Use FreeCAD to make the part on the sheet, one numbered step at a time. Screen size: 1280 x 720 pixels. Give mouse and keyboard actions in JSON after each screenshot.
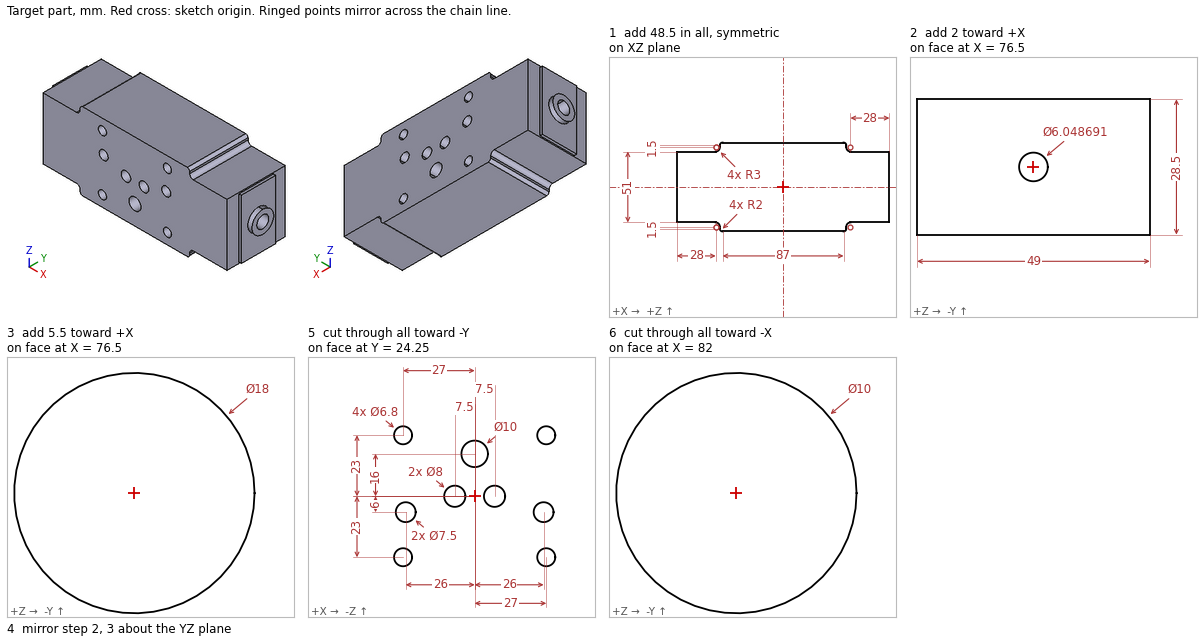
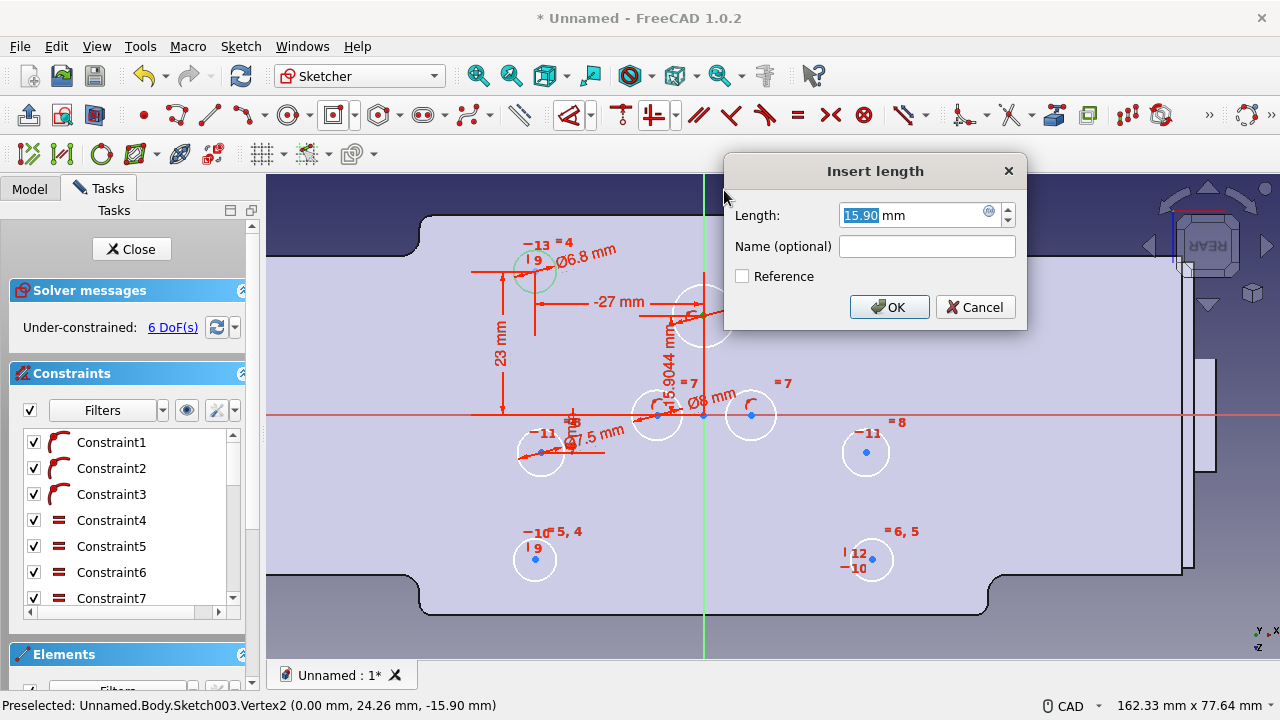
{"action": "type", "text": "16"}
{"action": "key", "text": "Return"}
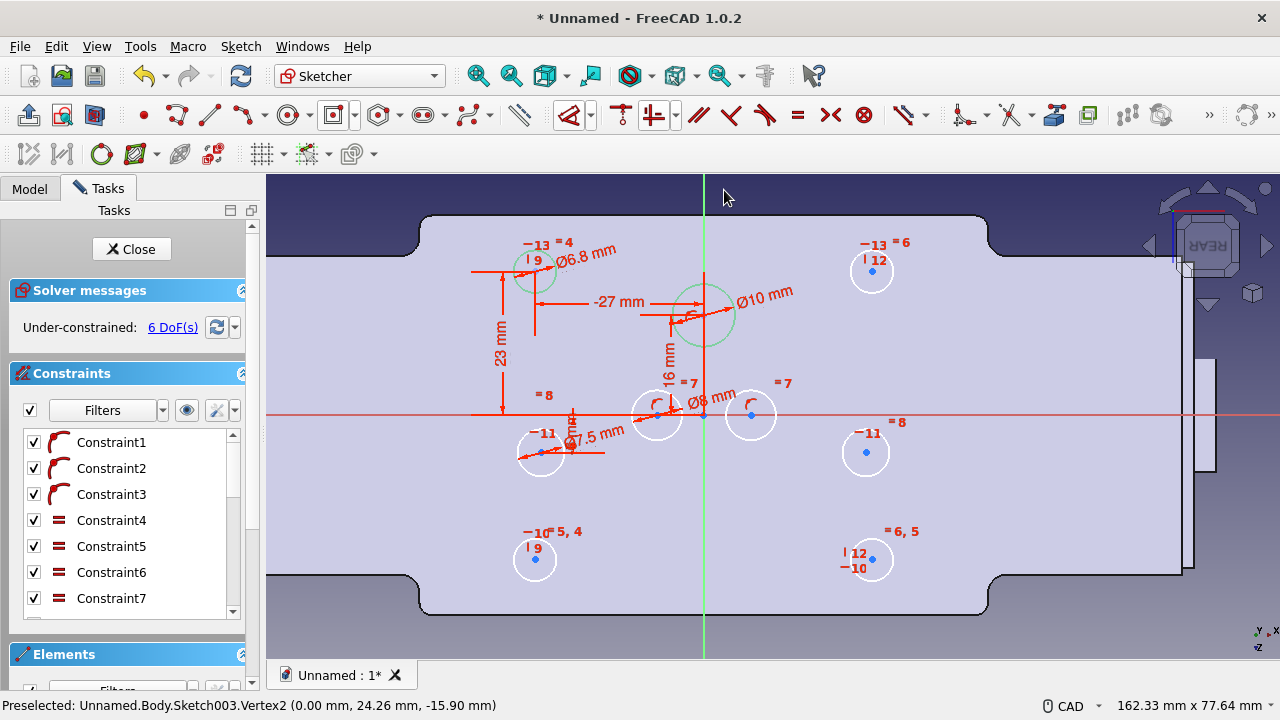
{"action": "left_click", "coordinate": [541, 453]}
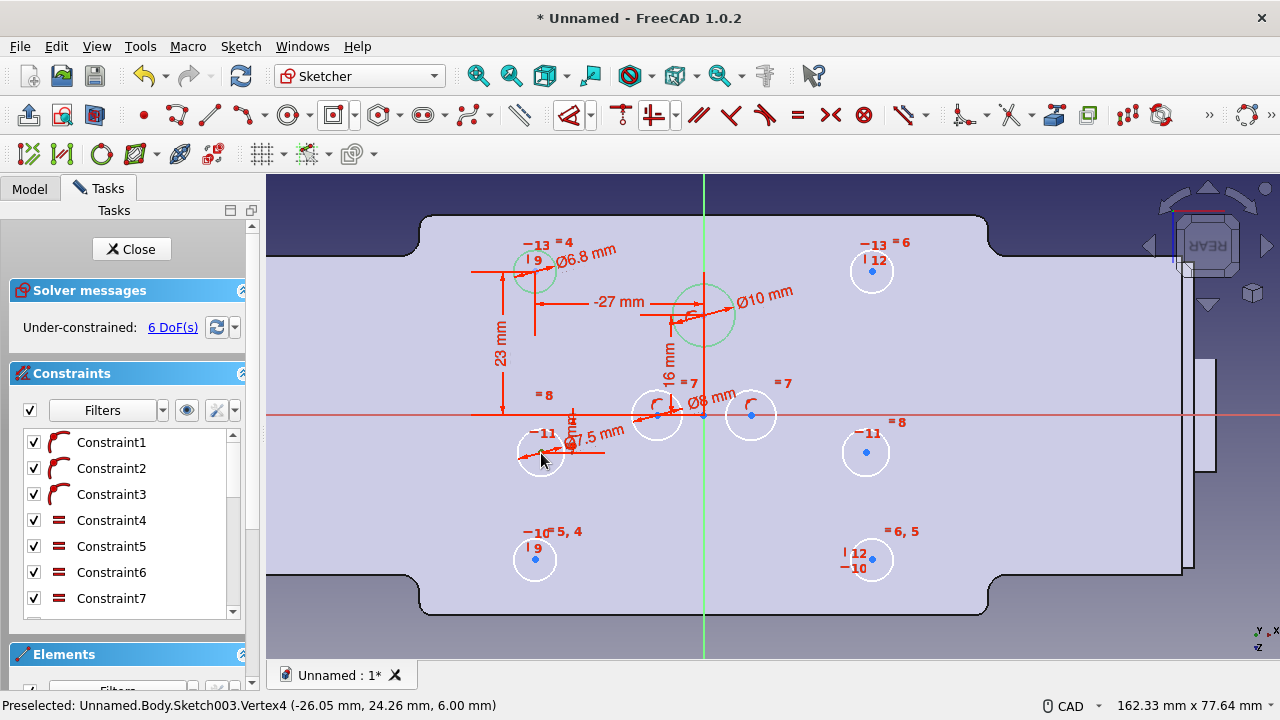
{"action": "left_click", "coordinate": [590, 116]}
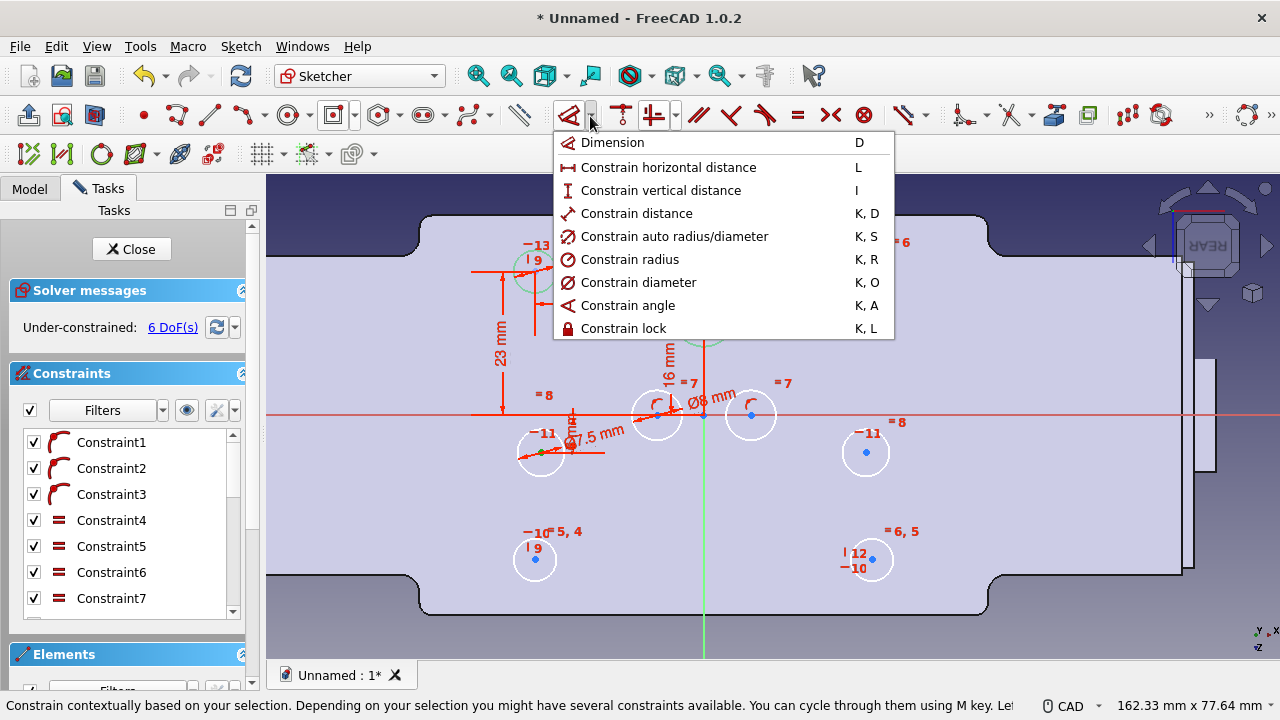
{"action": "left_click", "coordinate": [724, 168]}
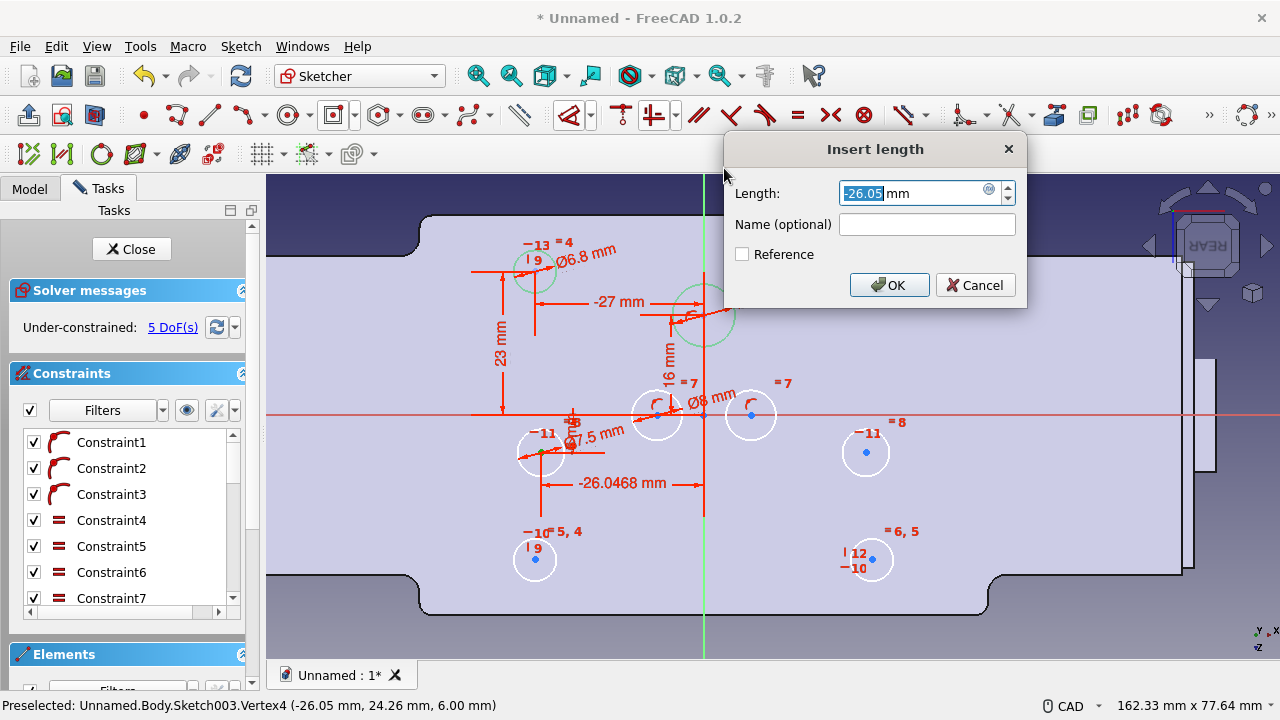
{"action": "type", "text": "-26"}
{"action": "key", "text": "Return"}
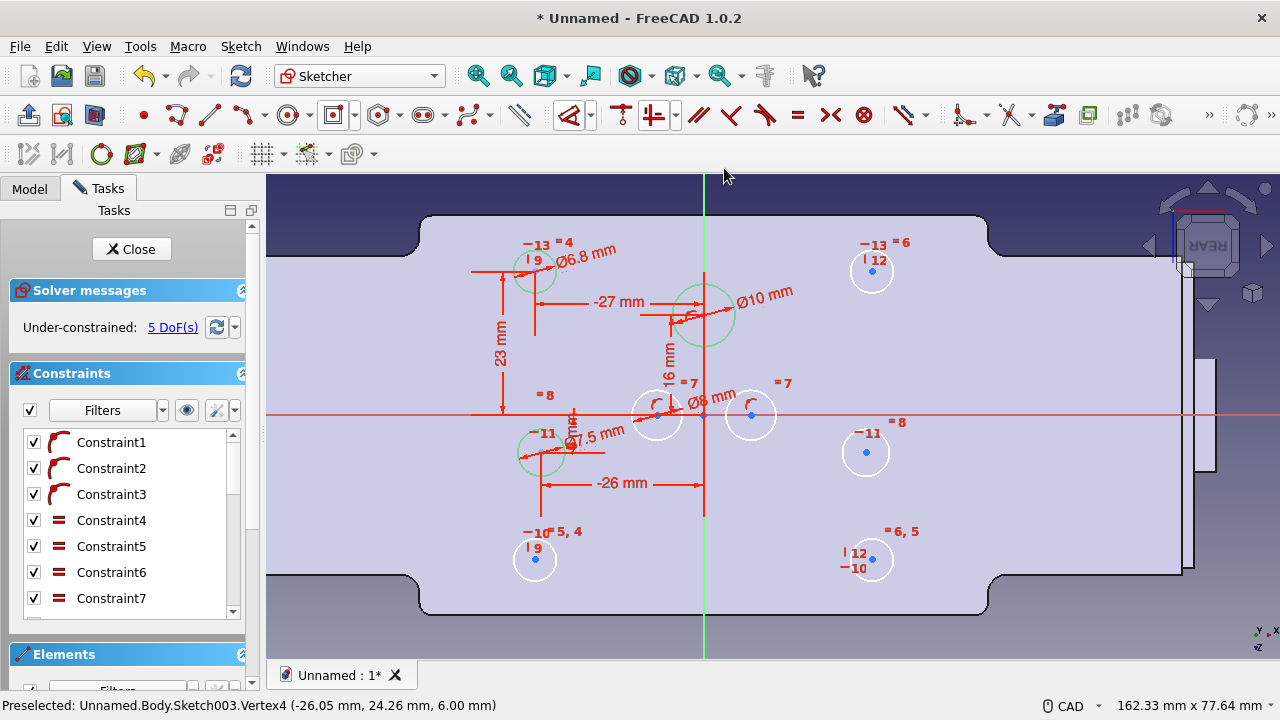
{"action": "left_click", "coordinate": [535, 560]}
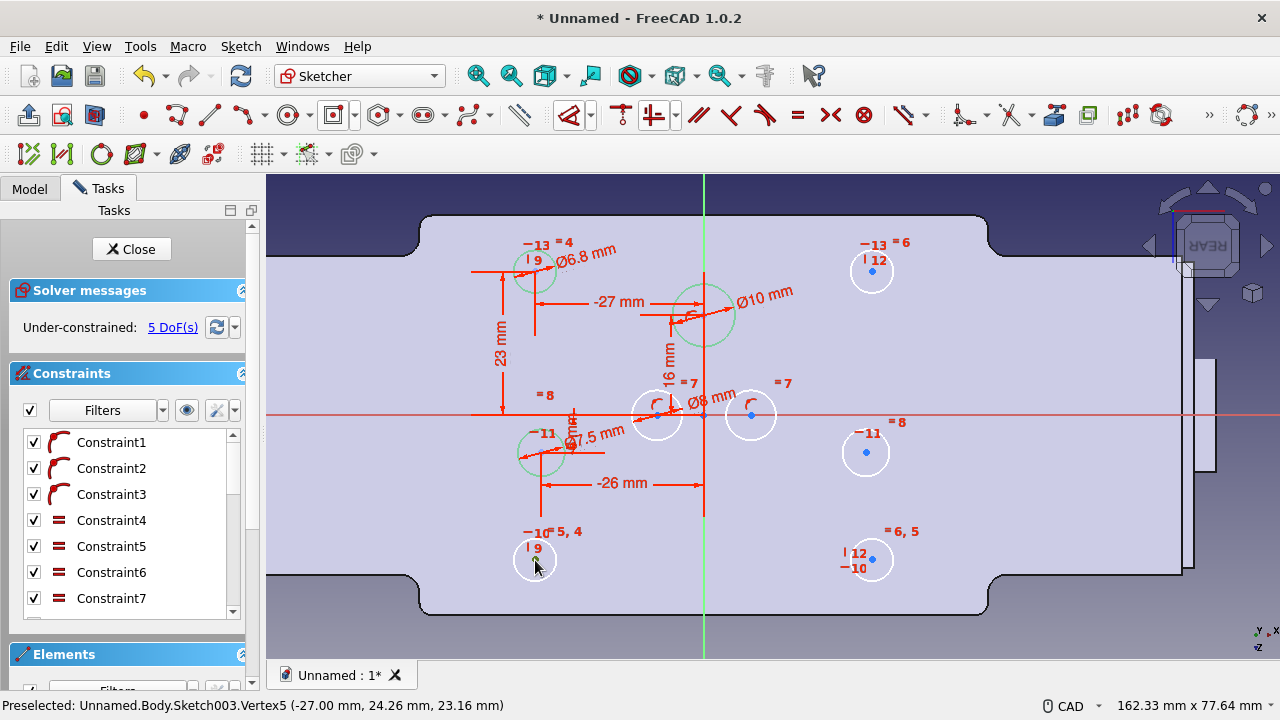
{"action": "left_click", "coordinate": [590, 116]}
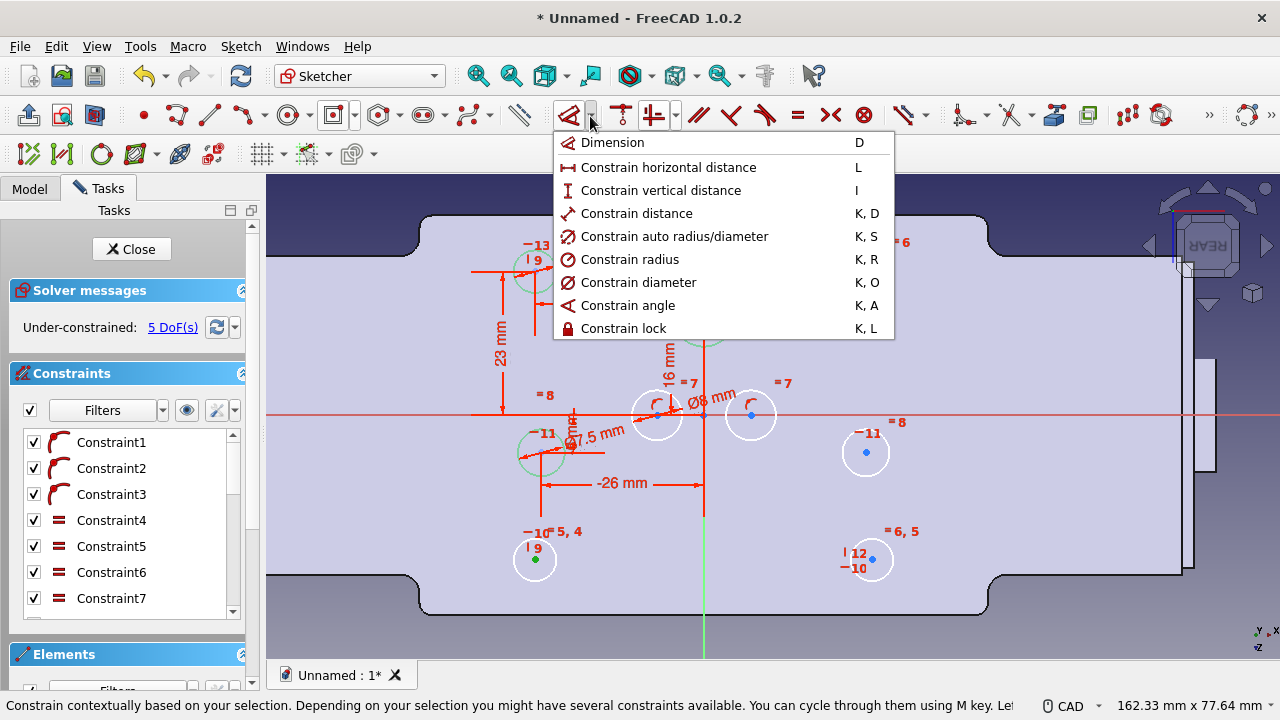
{"action": "left_click", "coordinate": [724, 190]}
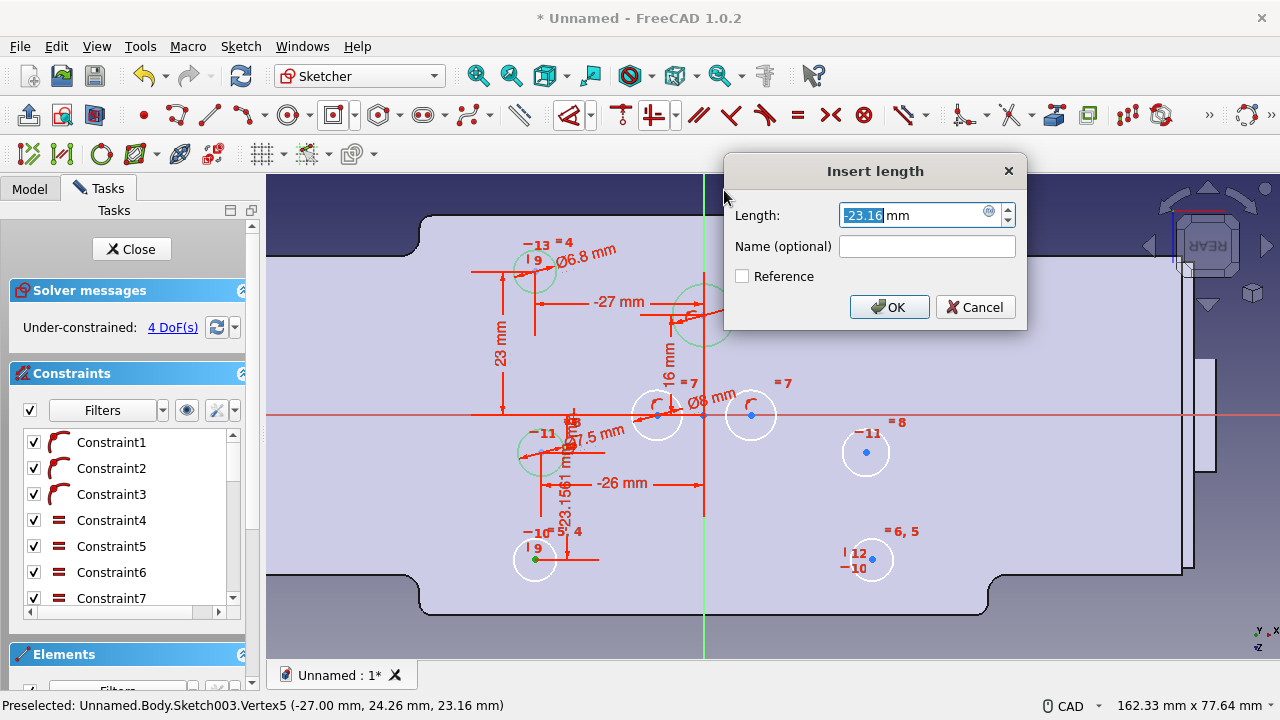
{"action": "type", "text": "-23"}
{"action": "key", "text": "Return"}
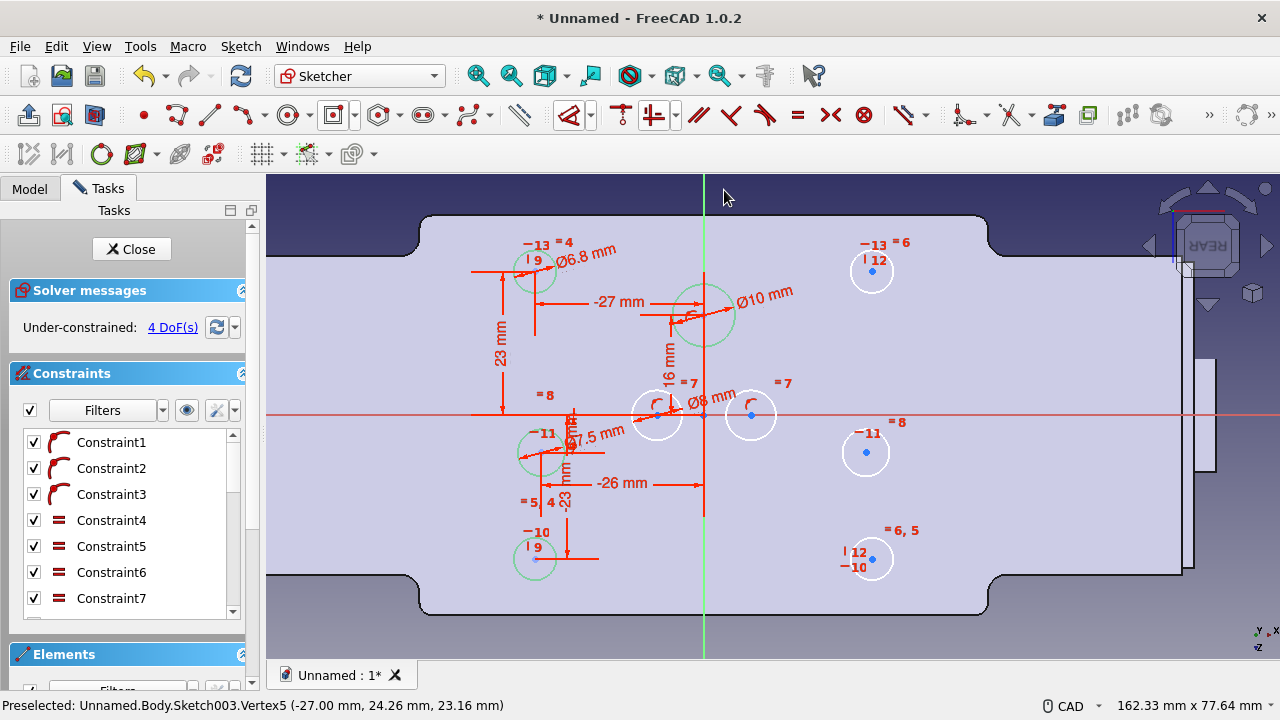
{"action": "left_click", "coordinate": [872, 559]}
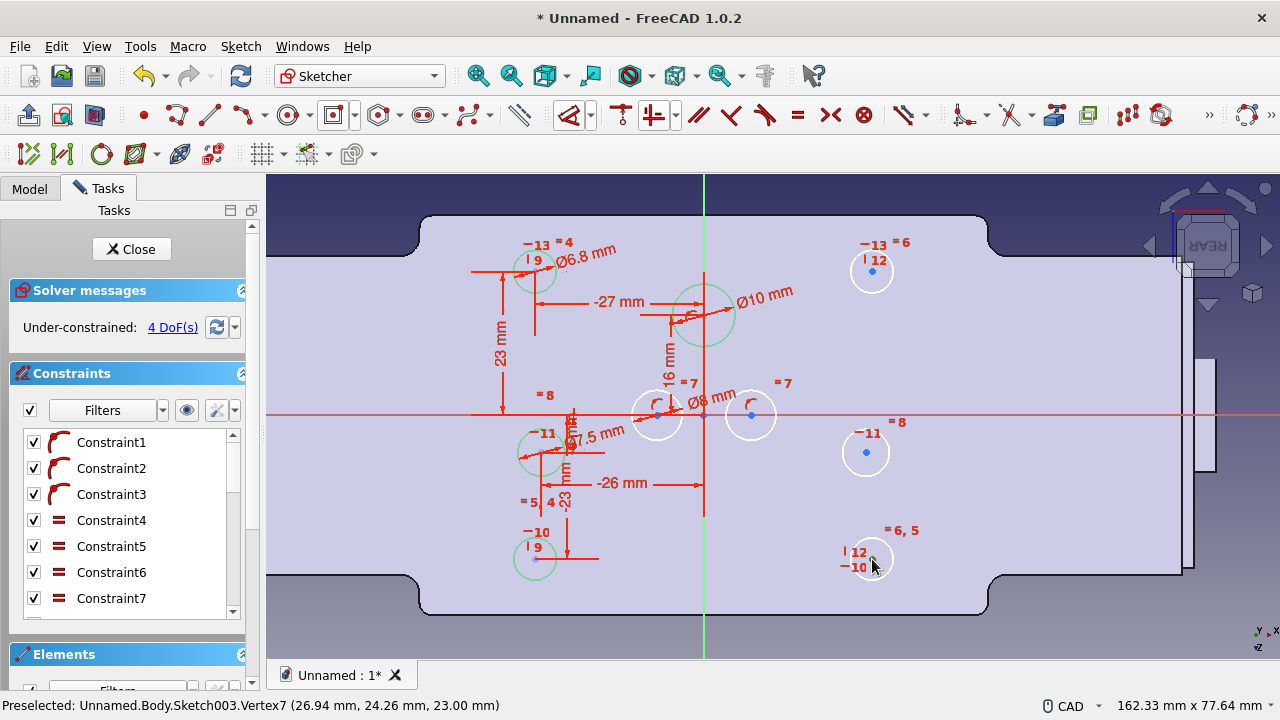
{"action": "key", "text": "l"}